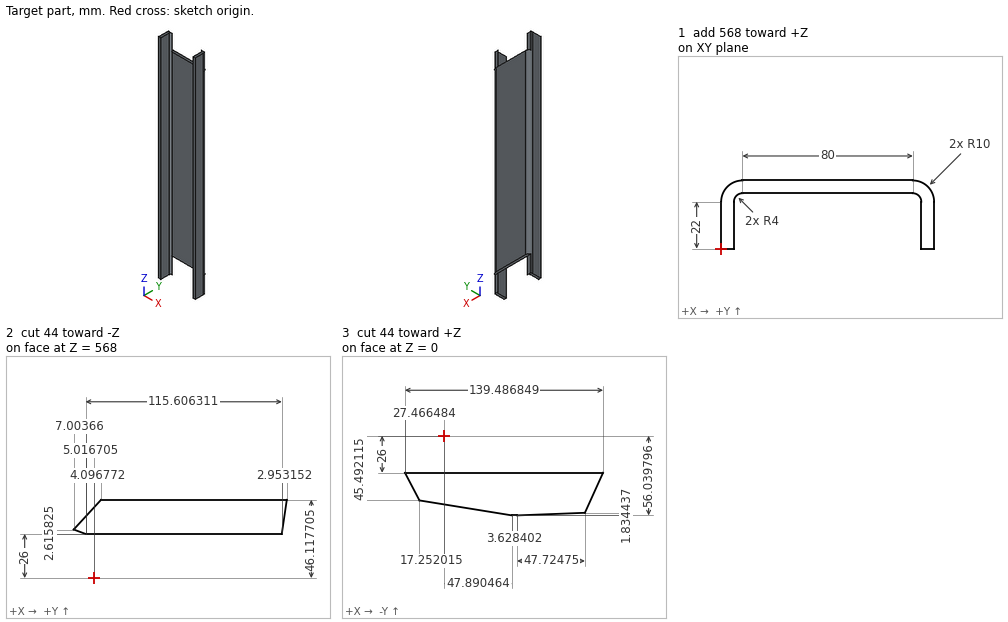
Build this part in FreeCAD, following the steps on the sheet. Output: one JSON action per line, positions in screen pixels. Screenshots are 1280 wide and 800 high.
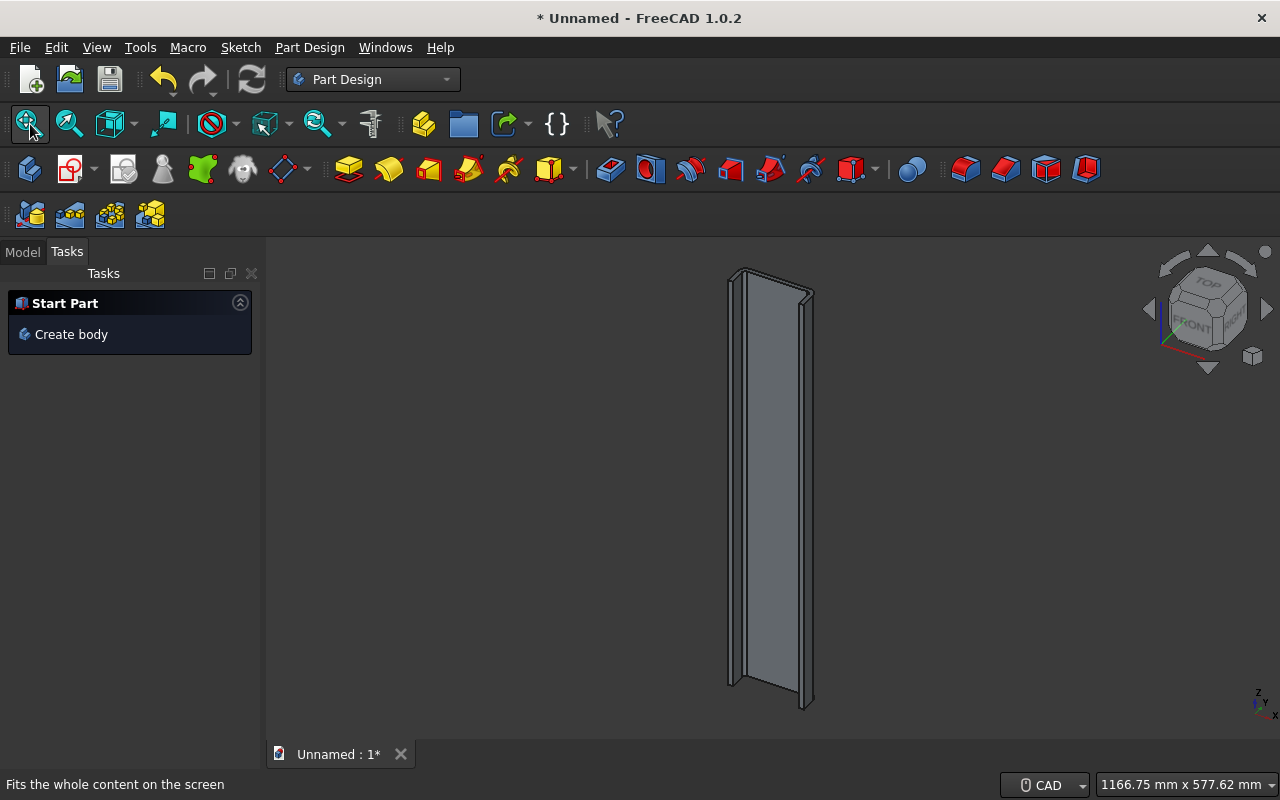
{"action": "scroll", "coordinate": [800, 286], "scroll_direction": "up", "scroll_amount": 9}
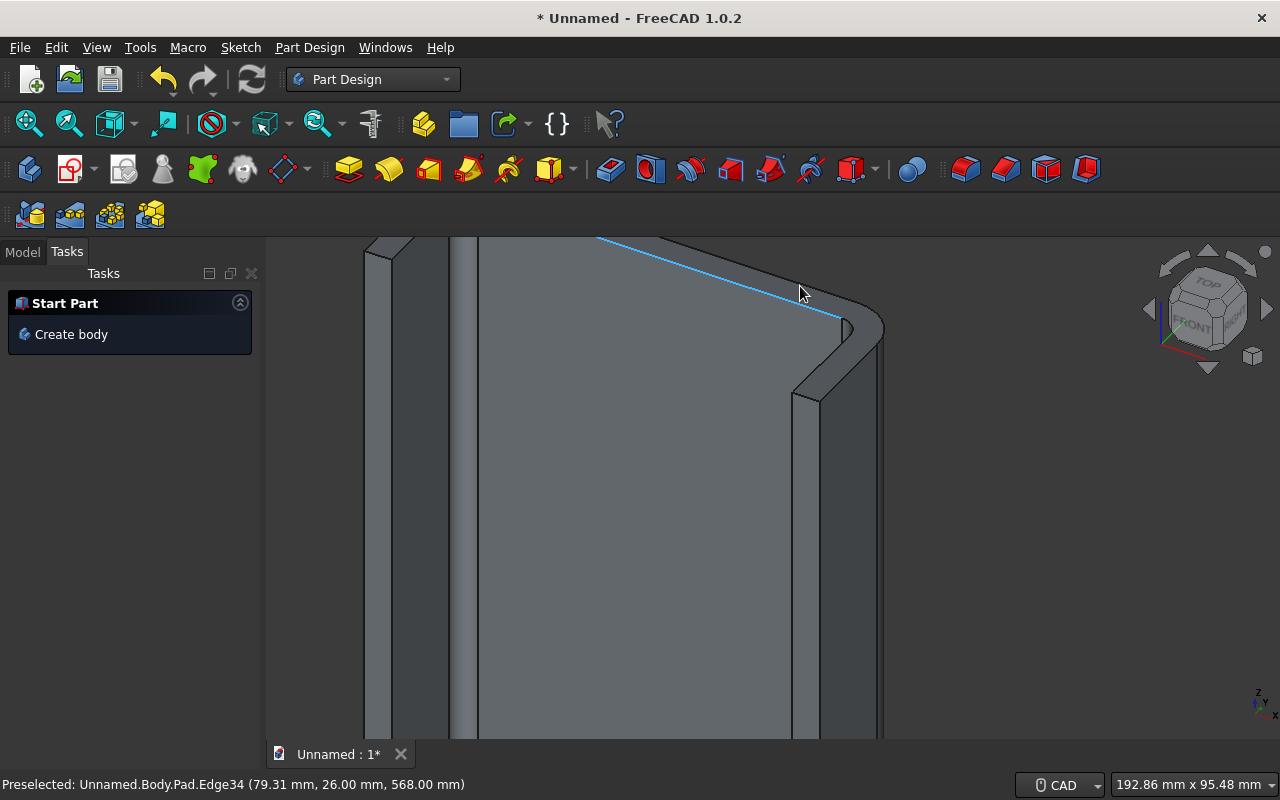
{"action": "left_click", "coordinate": [800, 291]}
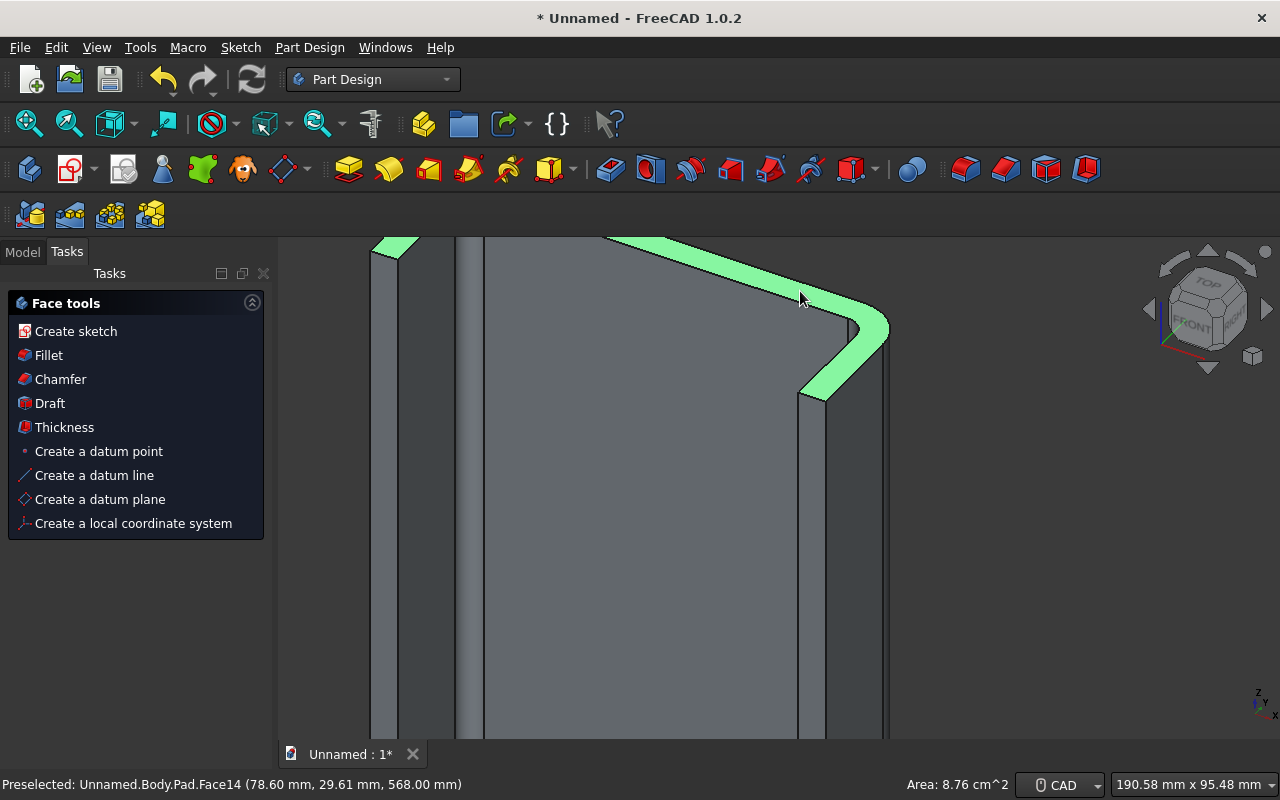
{"action": "left_click", "coordinate": [70, 170]}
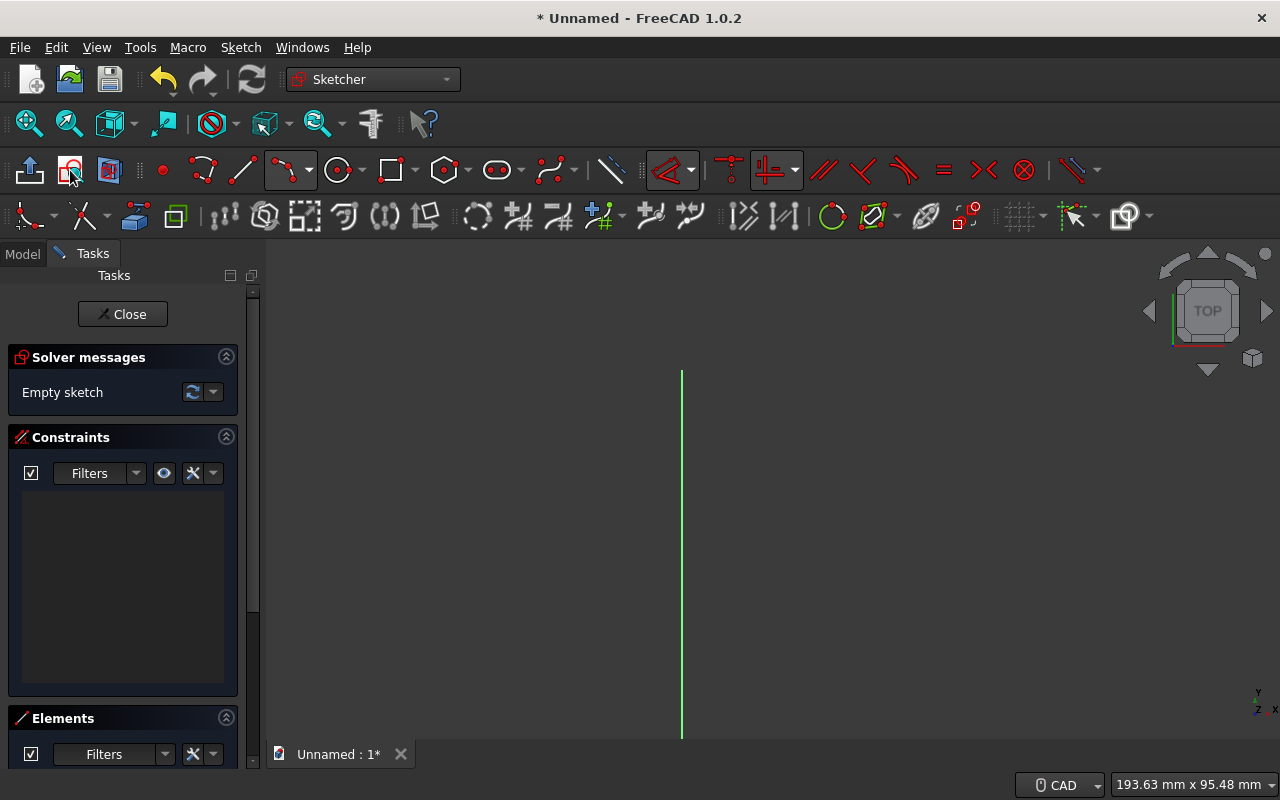
{"action": "scroll", "coordinate": [506, 267], "scroll_direction": "down", "scroll_amount": 4}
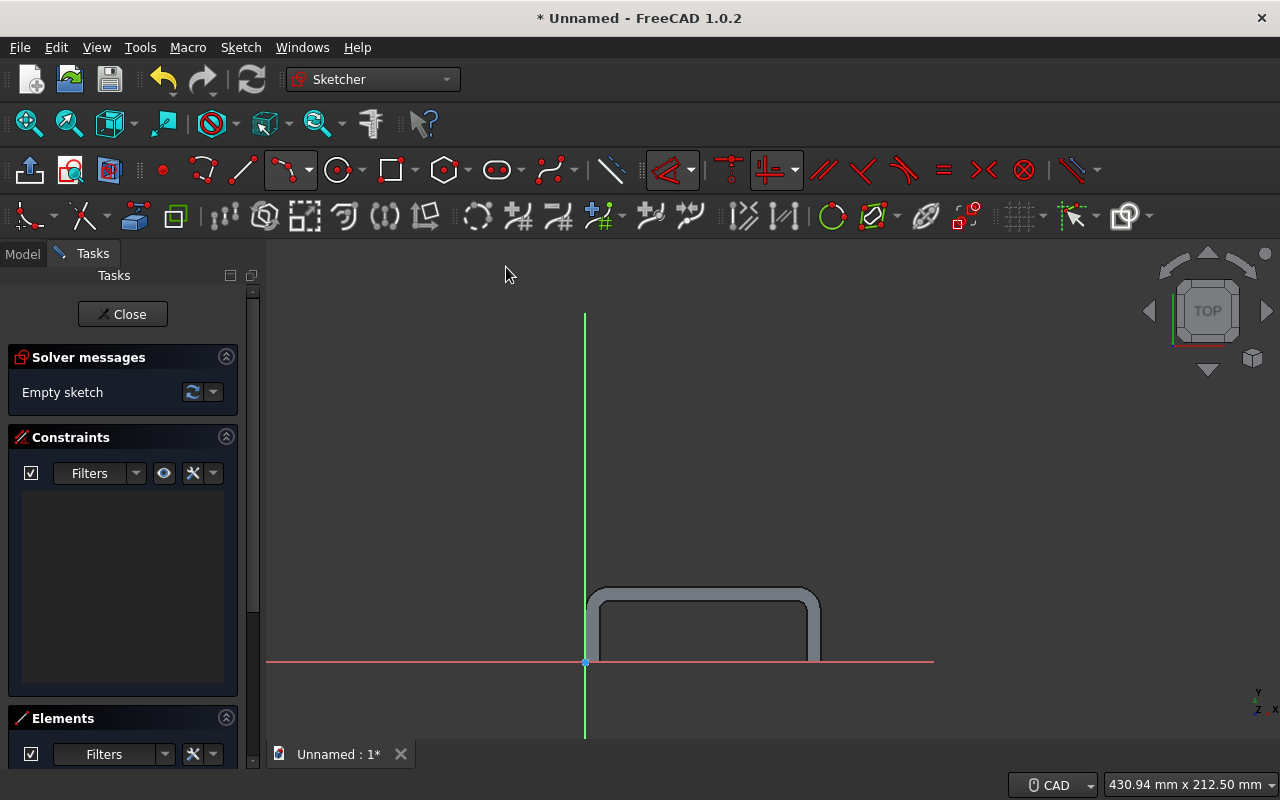
{"action": "scroll", "coordinate": [705, 711], "scroll_direction": "up", "scroll_amount": 3}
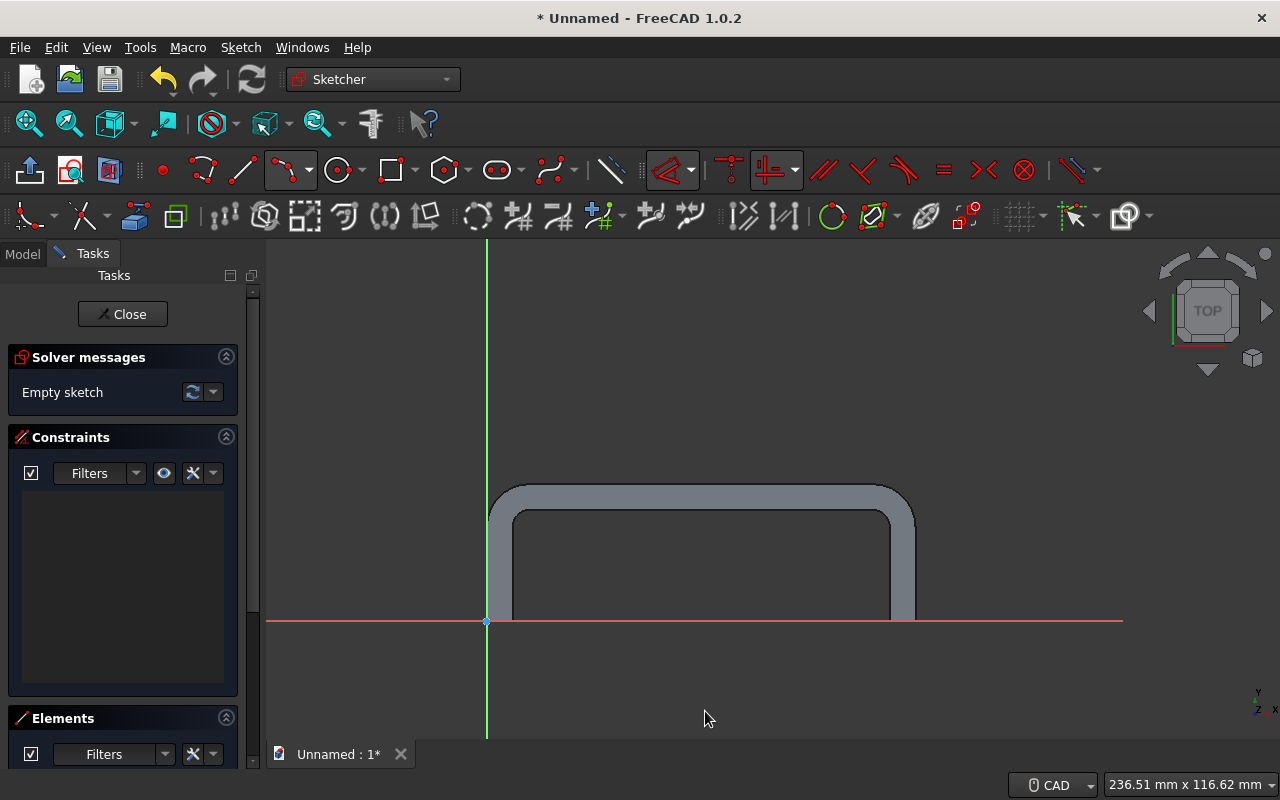
{"action": "left_click", "coordinate": [204, 170]}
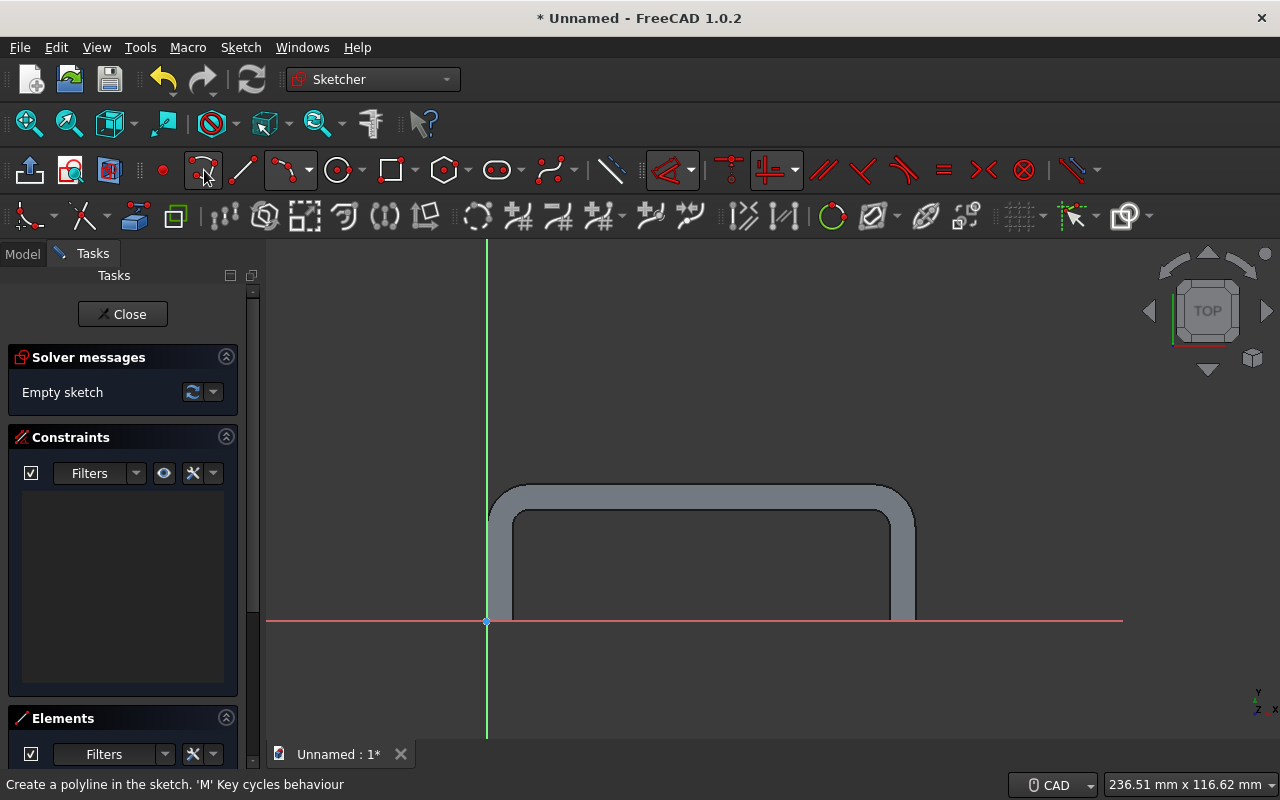
{"action": "left_click", "coordinate": [465, 510]}
{"action": "left_click", "coordinate": [961, 510]}
{"action": "left_click", "coordinate": [974, 424]}
{"action": "left_click", "coordinate": [504, 424]}
{"action": "left_click", "coordinate": [435, 499]}
{"action": "left_click", "coordinate": [465, 511]}
{"action": "key", "text": "Escape"}
{"action": "key", "text": "Escape"}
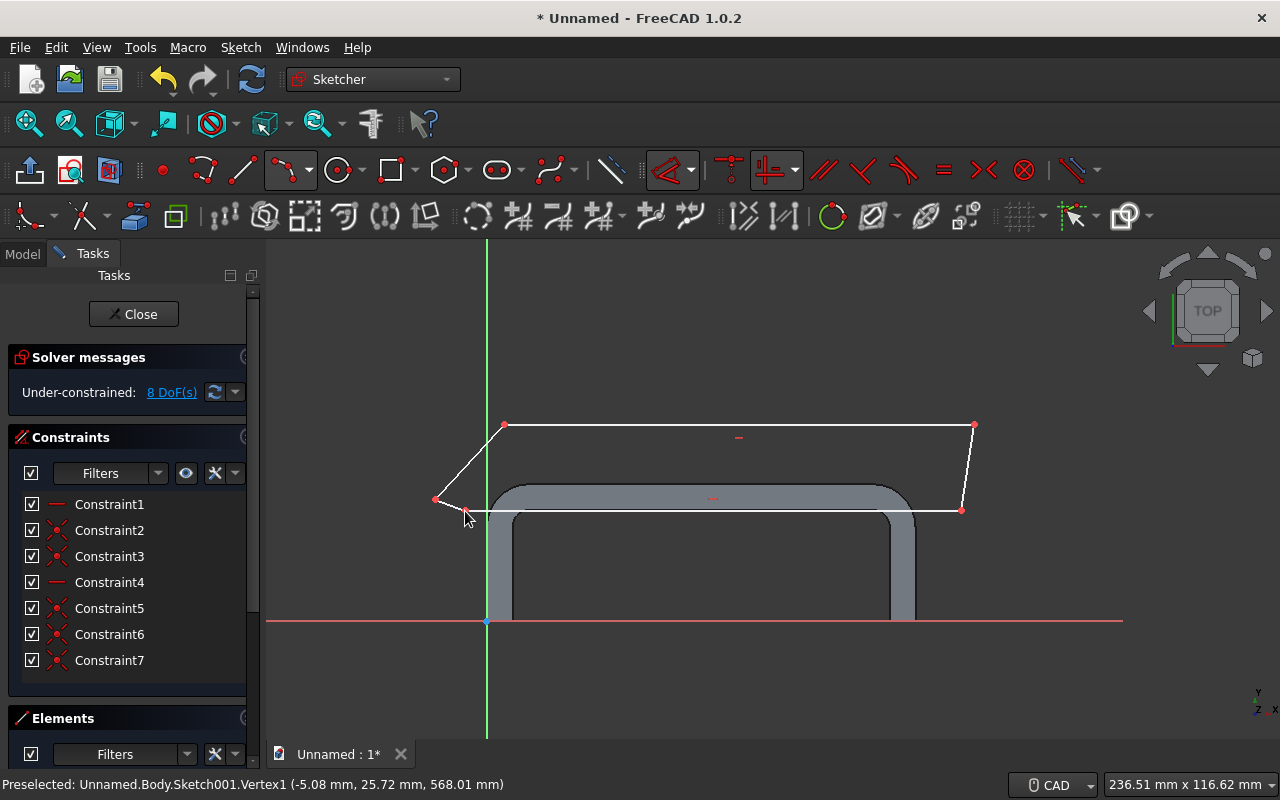
{"action": "left_click", "coordinate": [465, 511]}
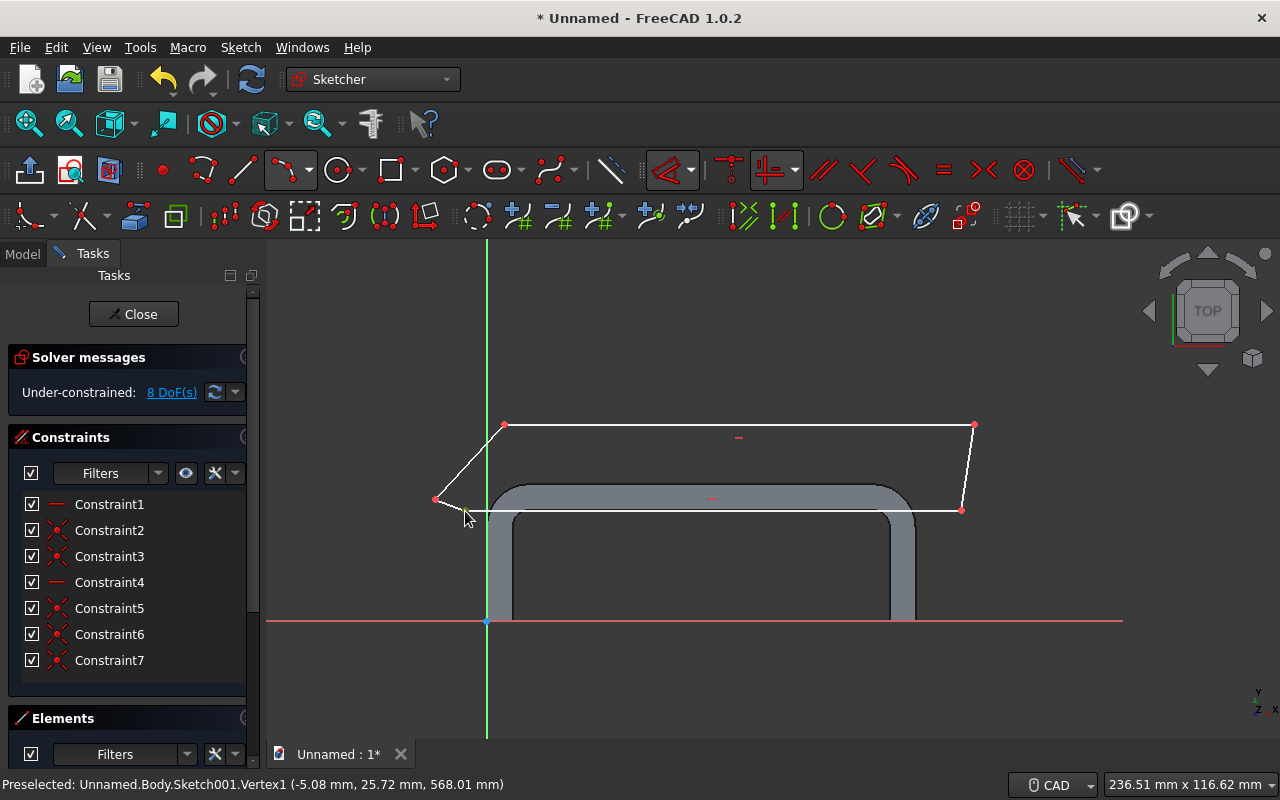
{"action": "left_click", "coordinate": [694, 170]}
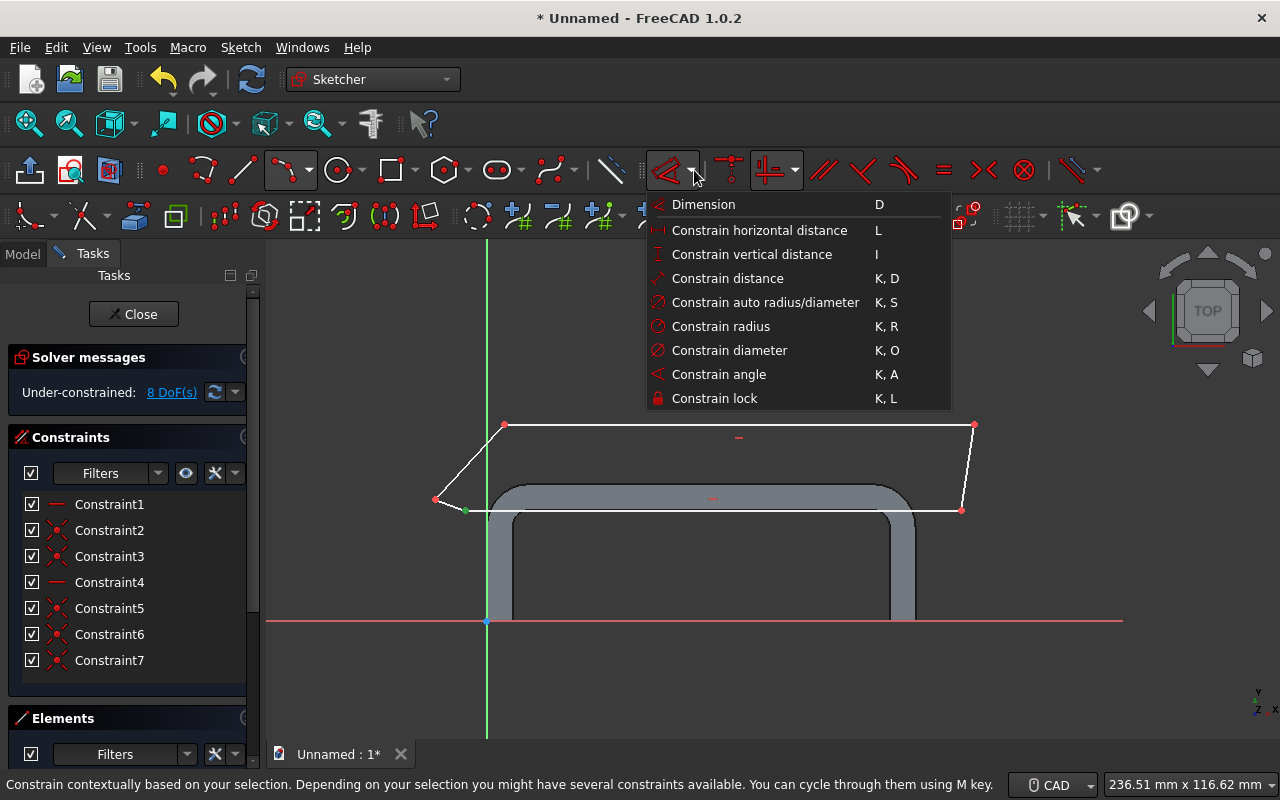
{"action": "left_click", "coordinate": [799, 254]}